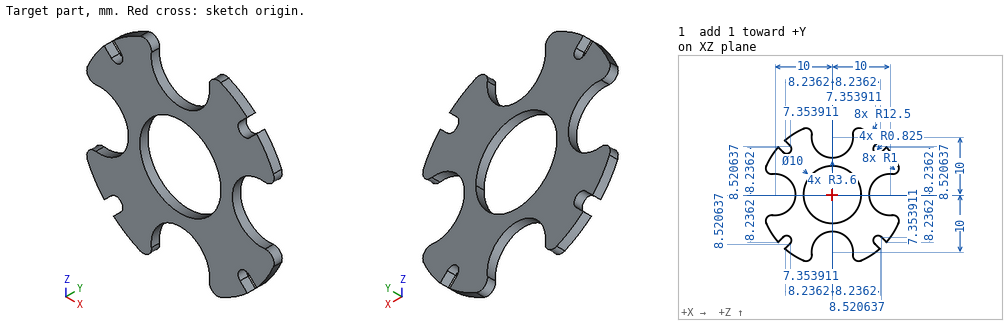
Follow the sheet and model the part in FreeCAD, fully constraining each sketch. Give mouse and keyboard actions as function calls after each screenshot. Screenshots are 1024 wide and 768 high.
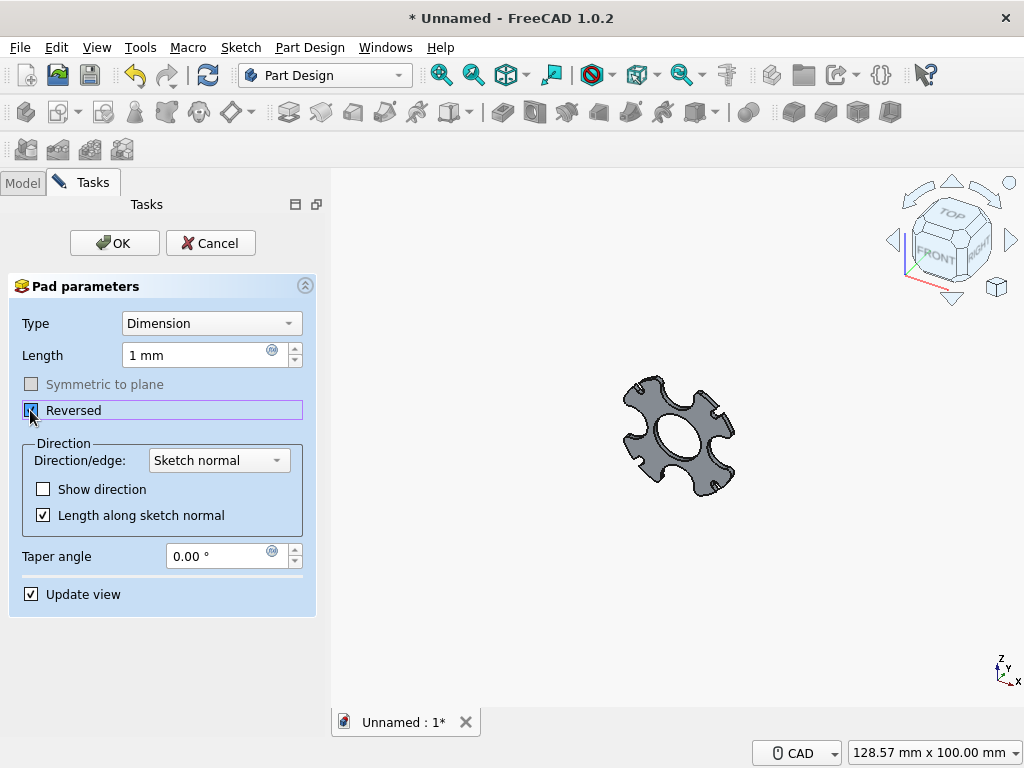
click(115, 243)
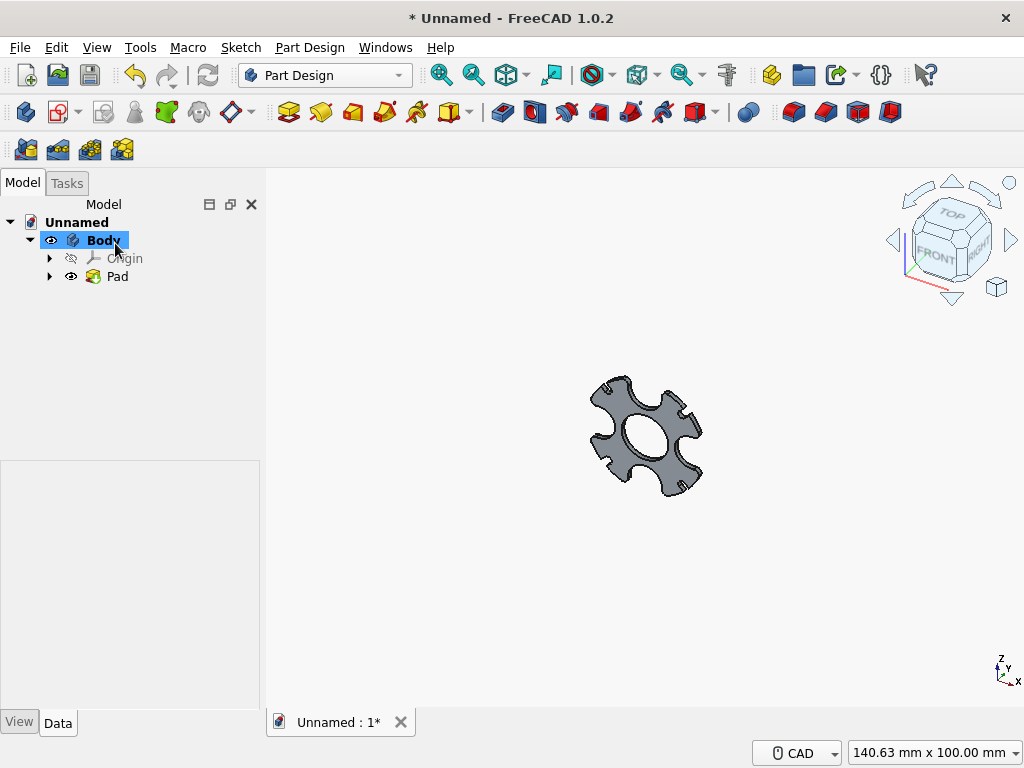
key(0)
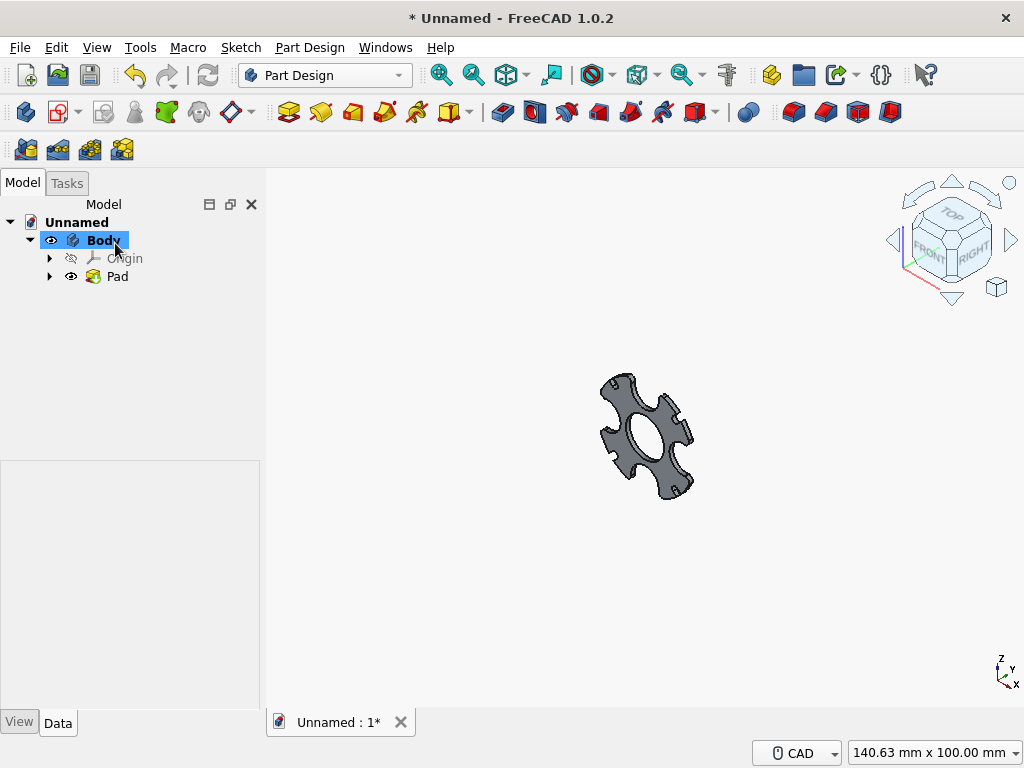
click(442, 76)